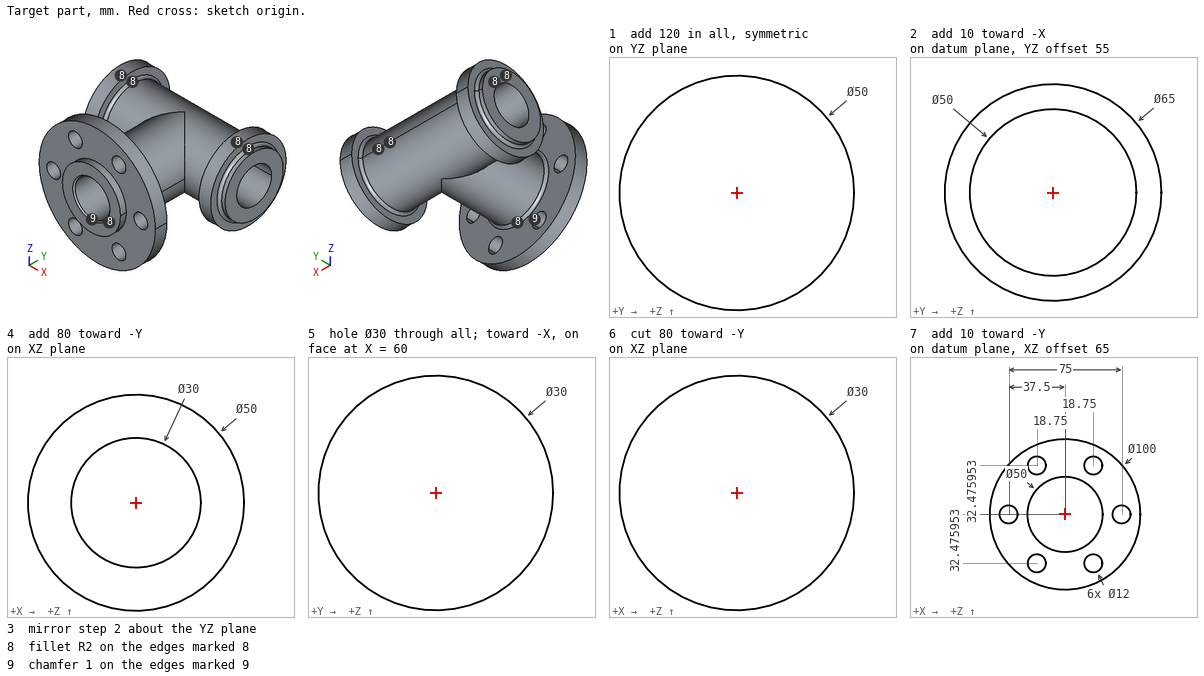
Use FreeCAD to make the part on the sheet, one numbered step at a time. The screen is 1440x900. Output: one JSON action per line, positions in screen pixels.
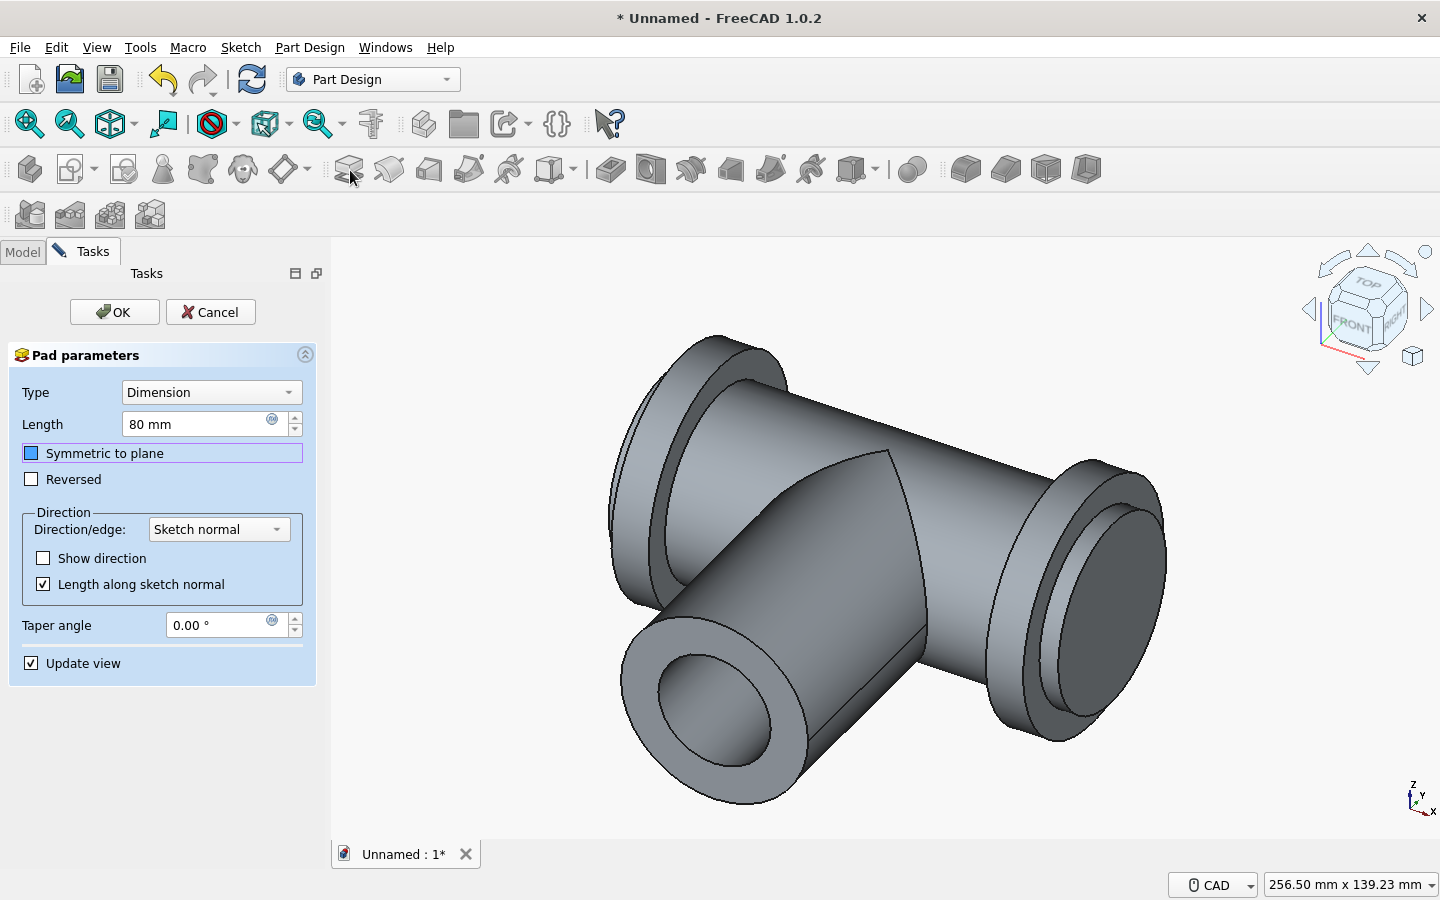
{"action": "left_click", "coordinate": [115, 312]}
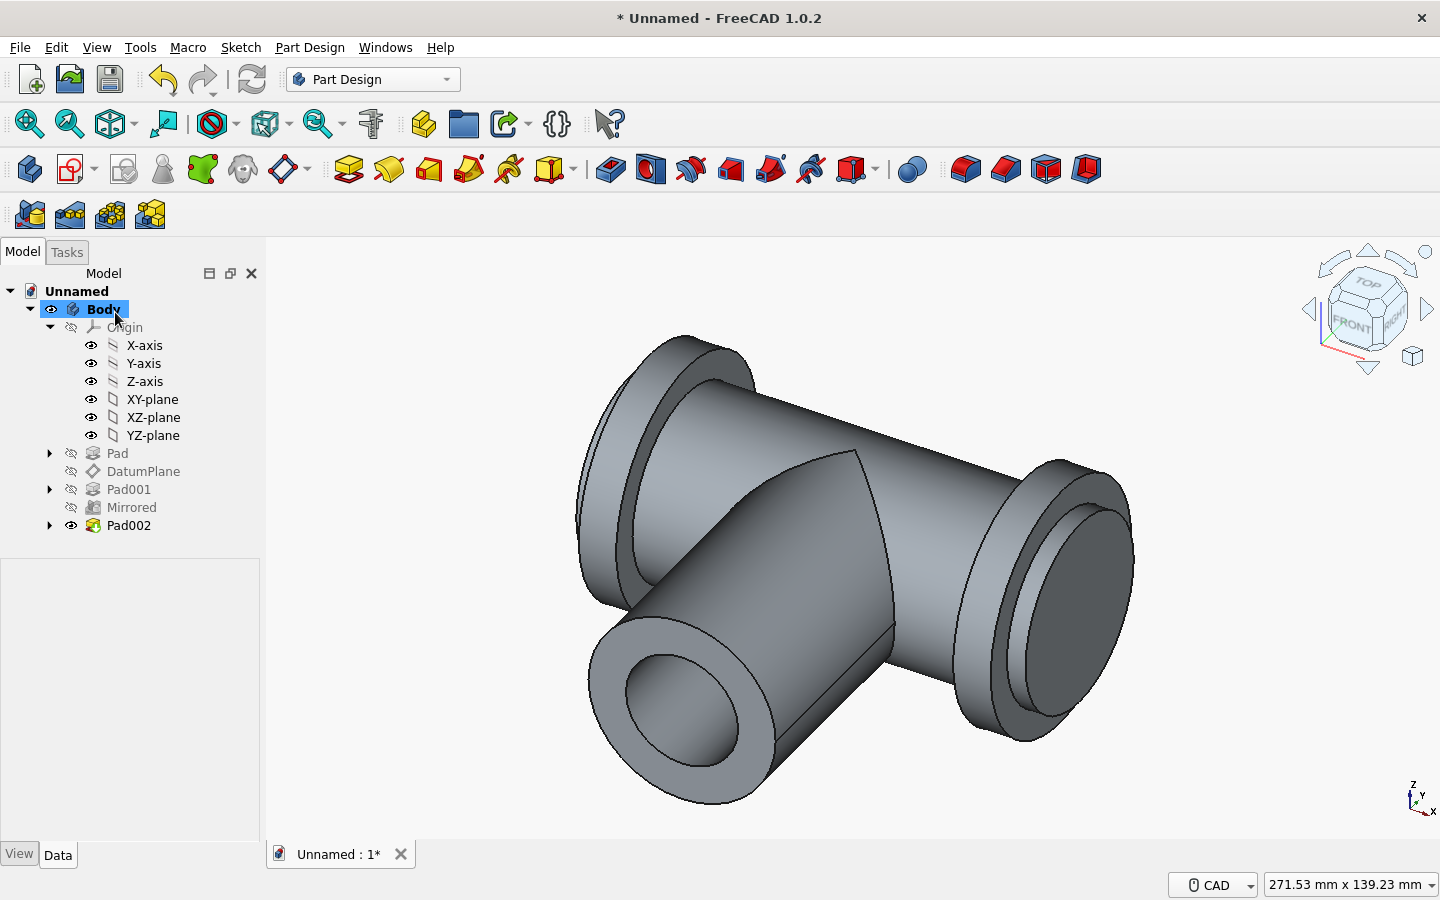
{"action": "left_click", "coordinate": [30, 124]}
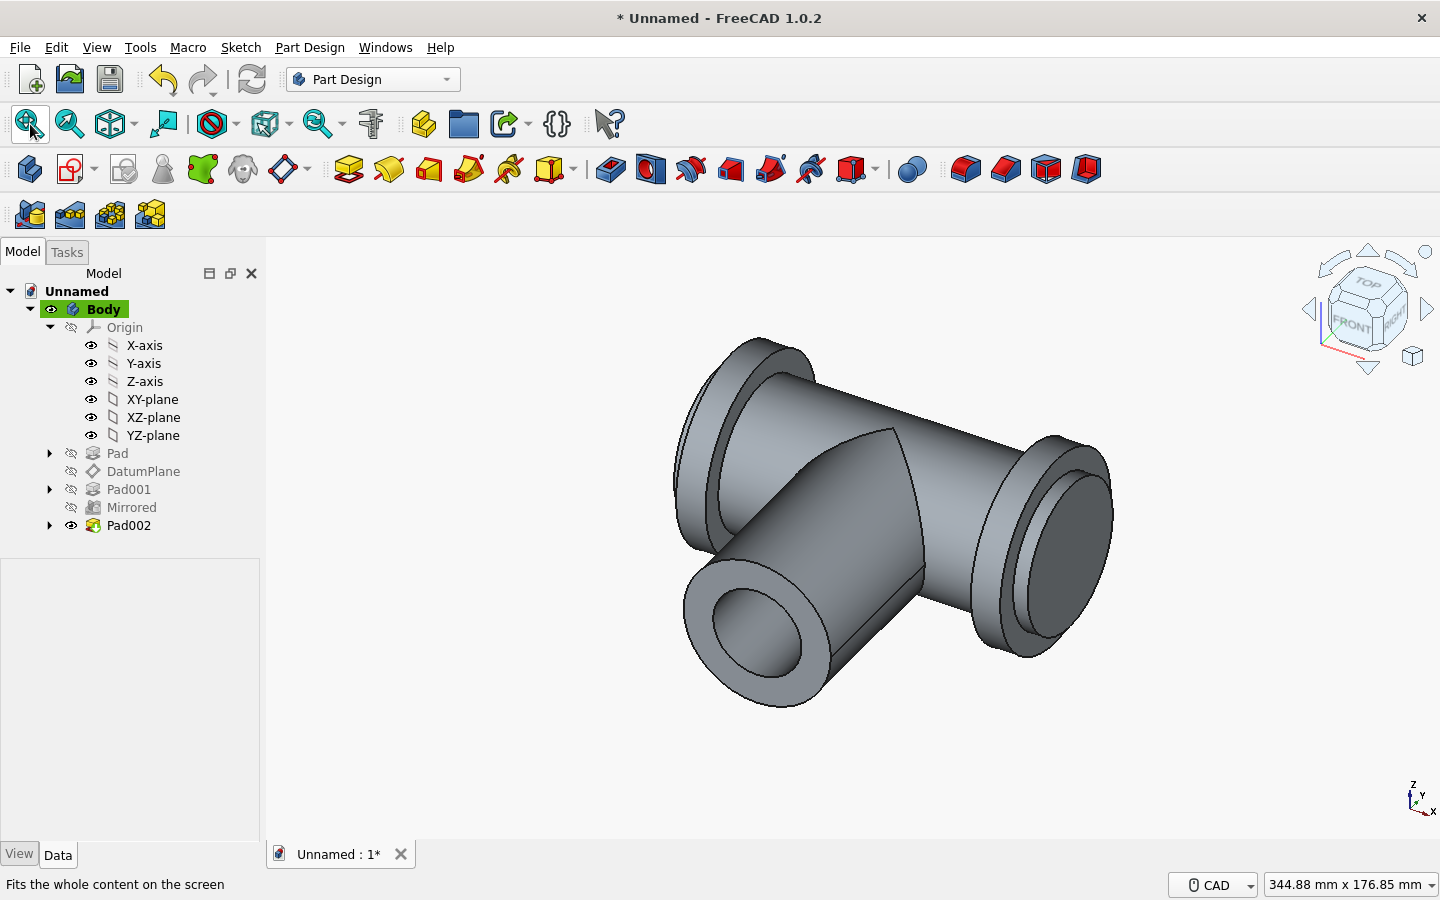
{"action": "left_click", "coordinate": [1070, 555]}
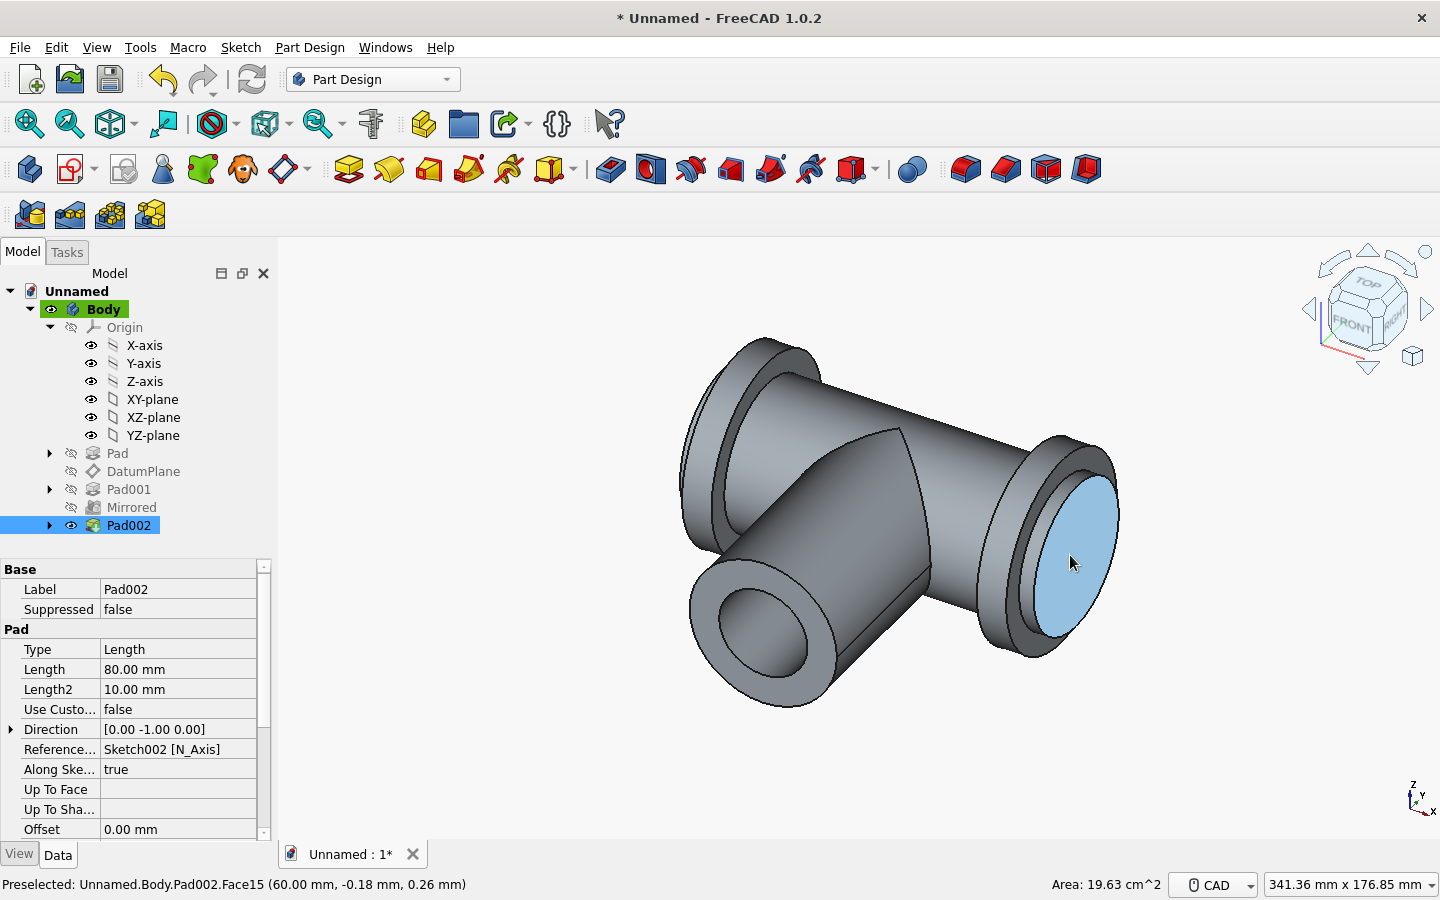
{"action": "left_click", "coordinate": [70, 170]}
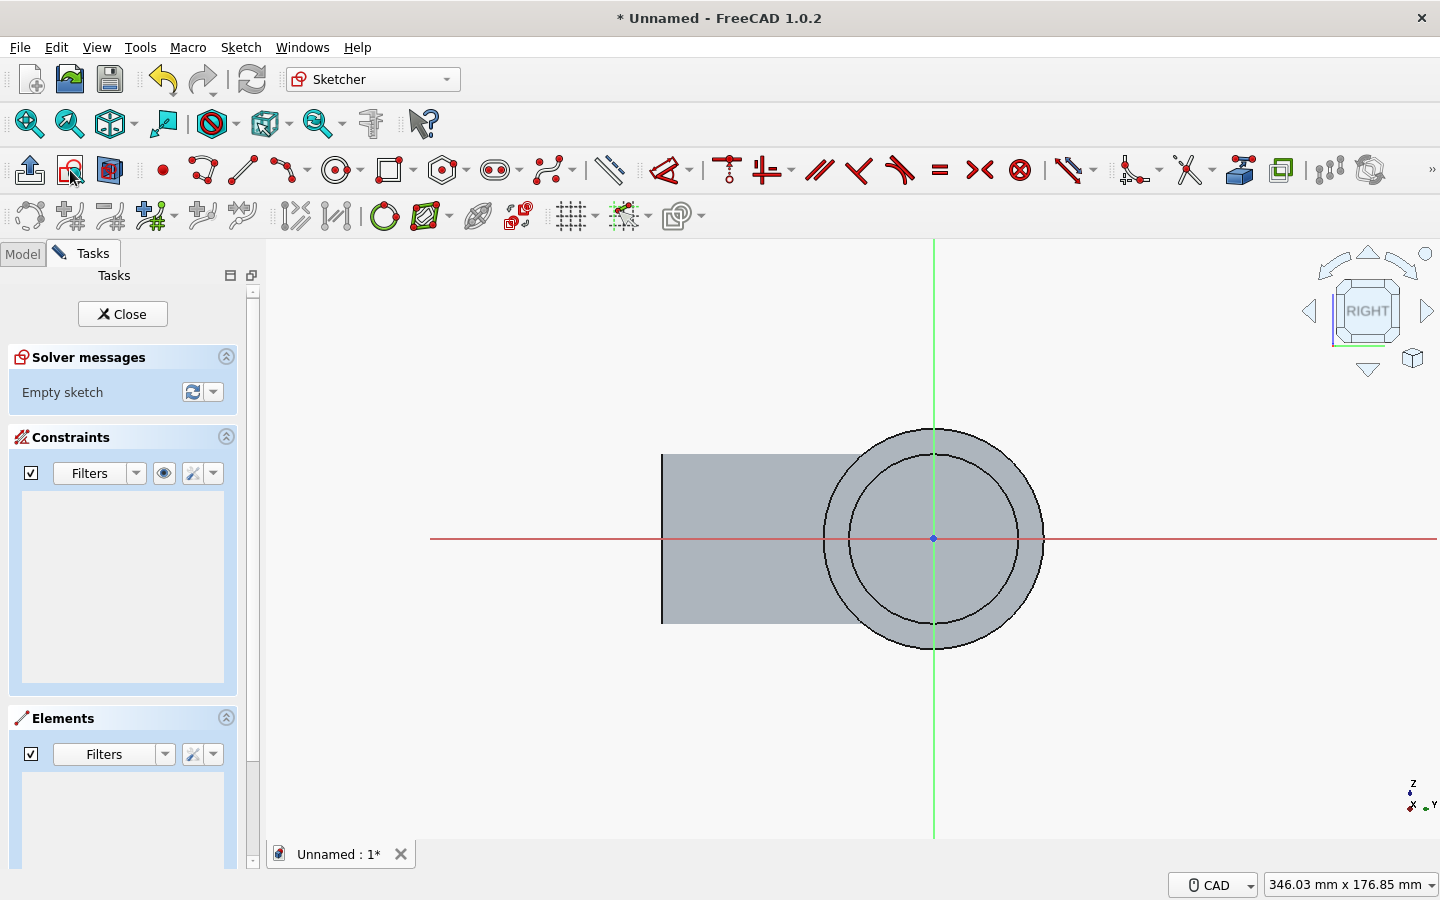
{"action": "scroll", "coordinate": [982, 539], "scroll_direction": "up", "scroll_amount": 7}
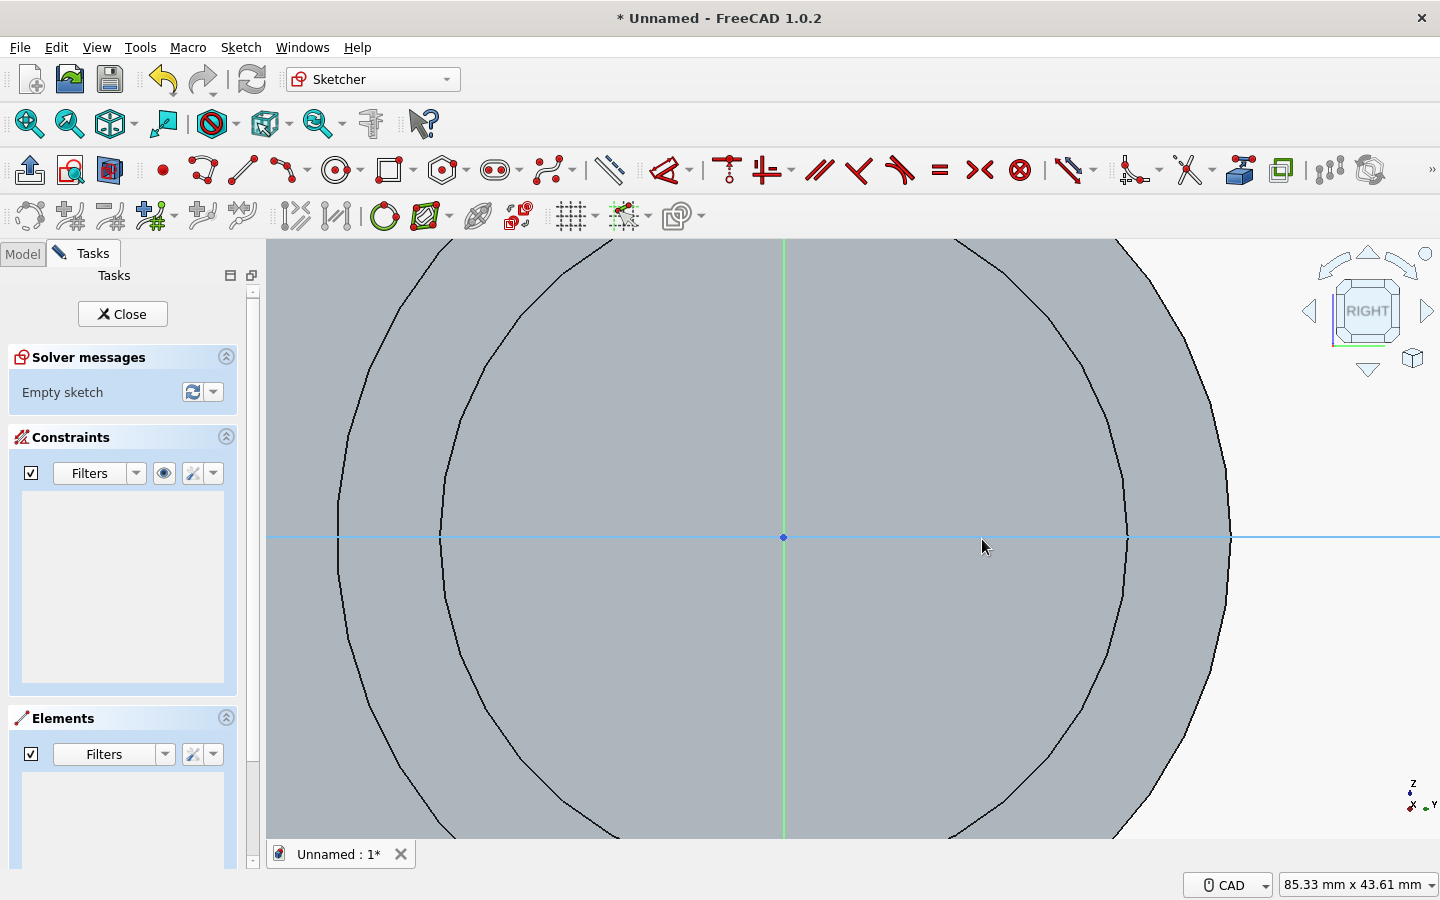
{"action": "key", "text": "g c"}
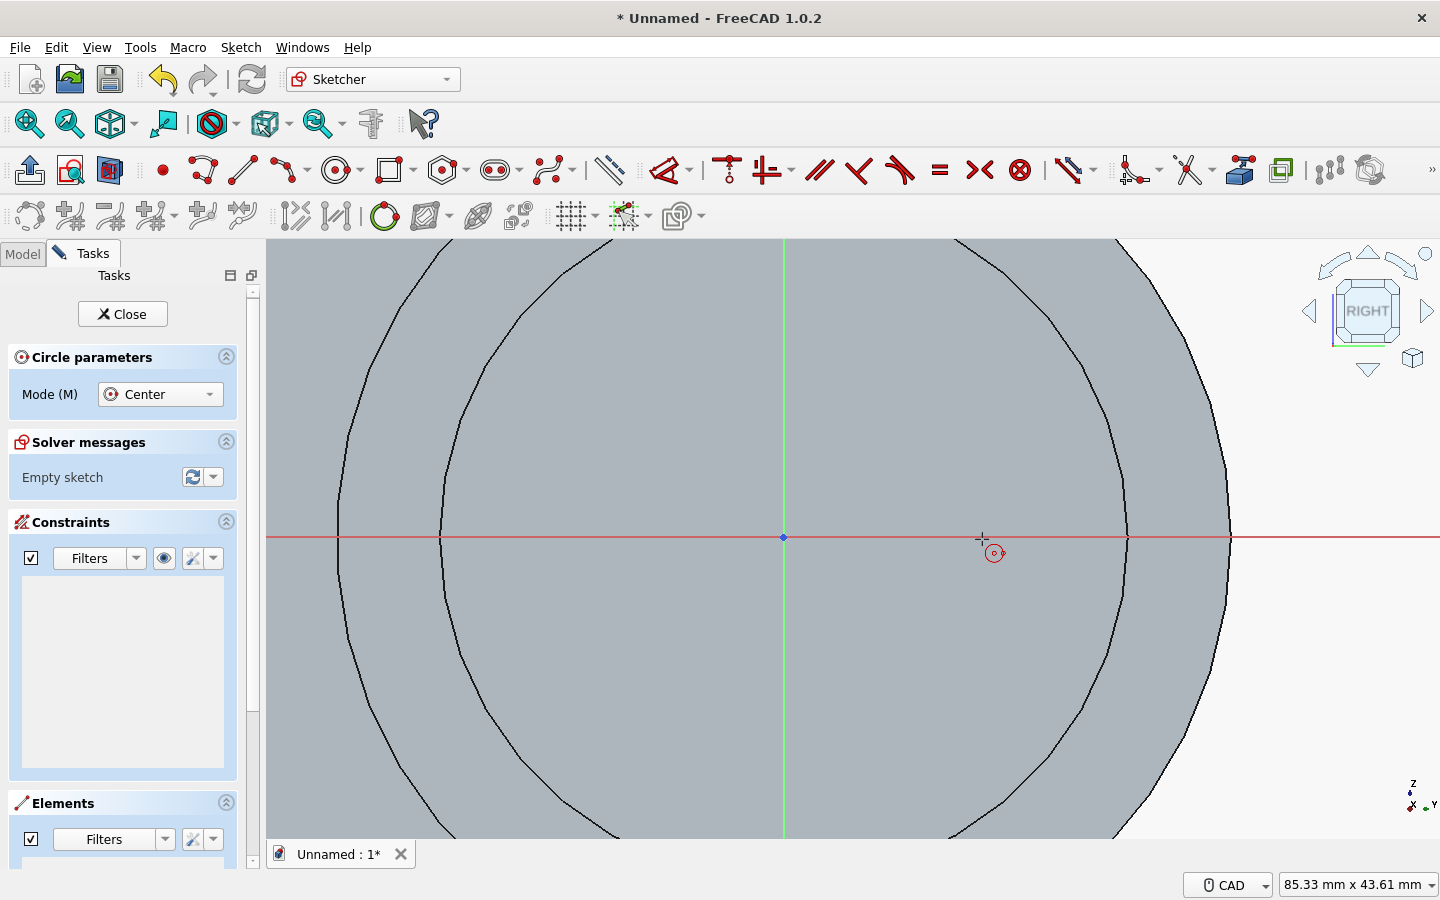
{"action": "left_click", "coordinate": [784, 537]}
{"action": "left_click", "coordinate": [930, 392]}
{"action": "key", "text": "Escape"}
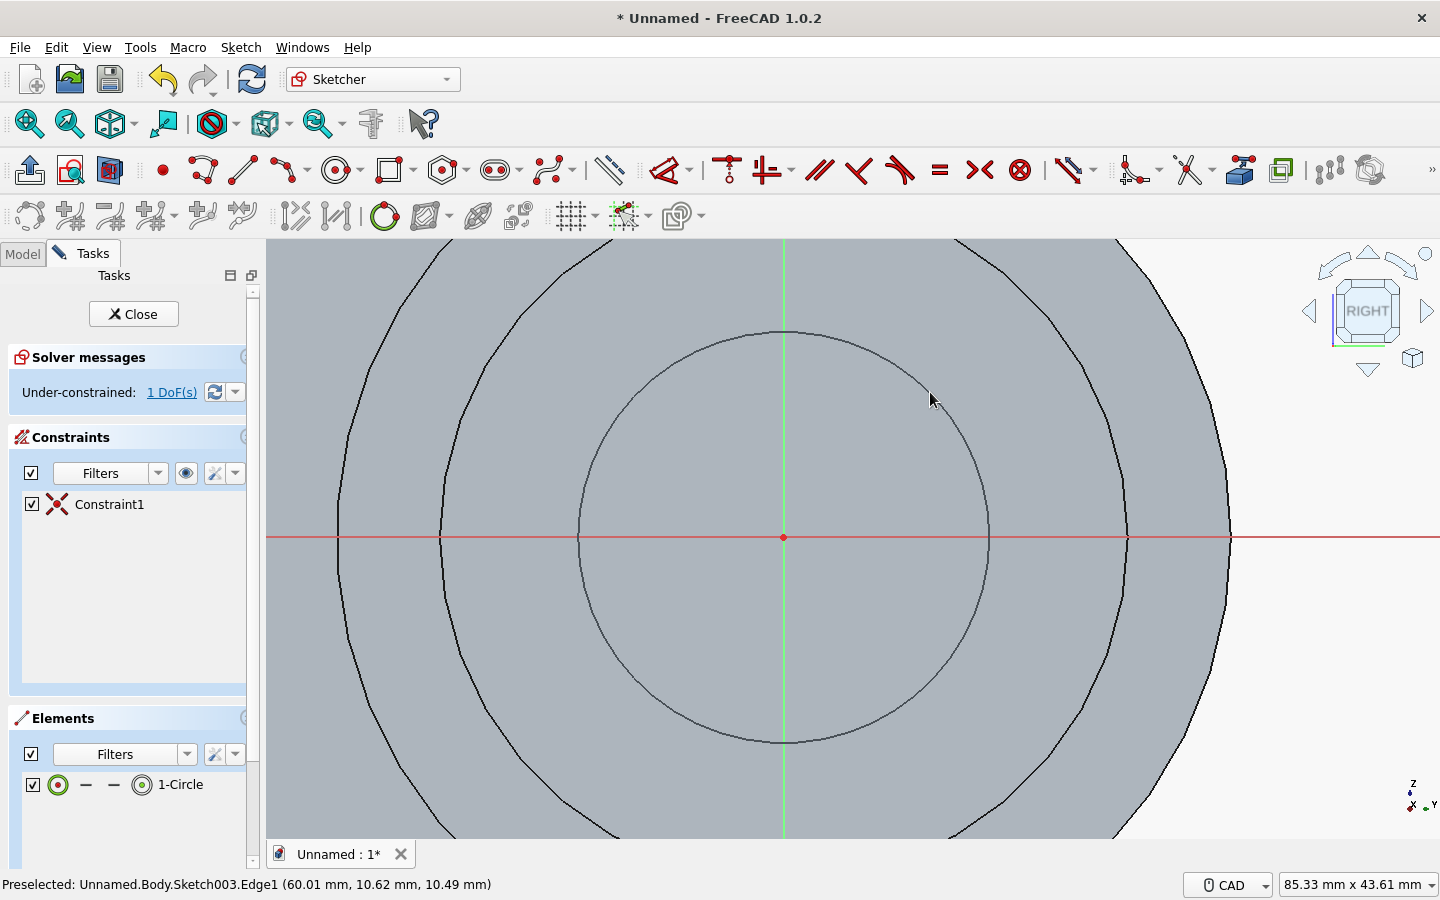
{"action": "left_click", "coordinate": [929, 392]}